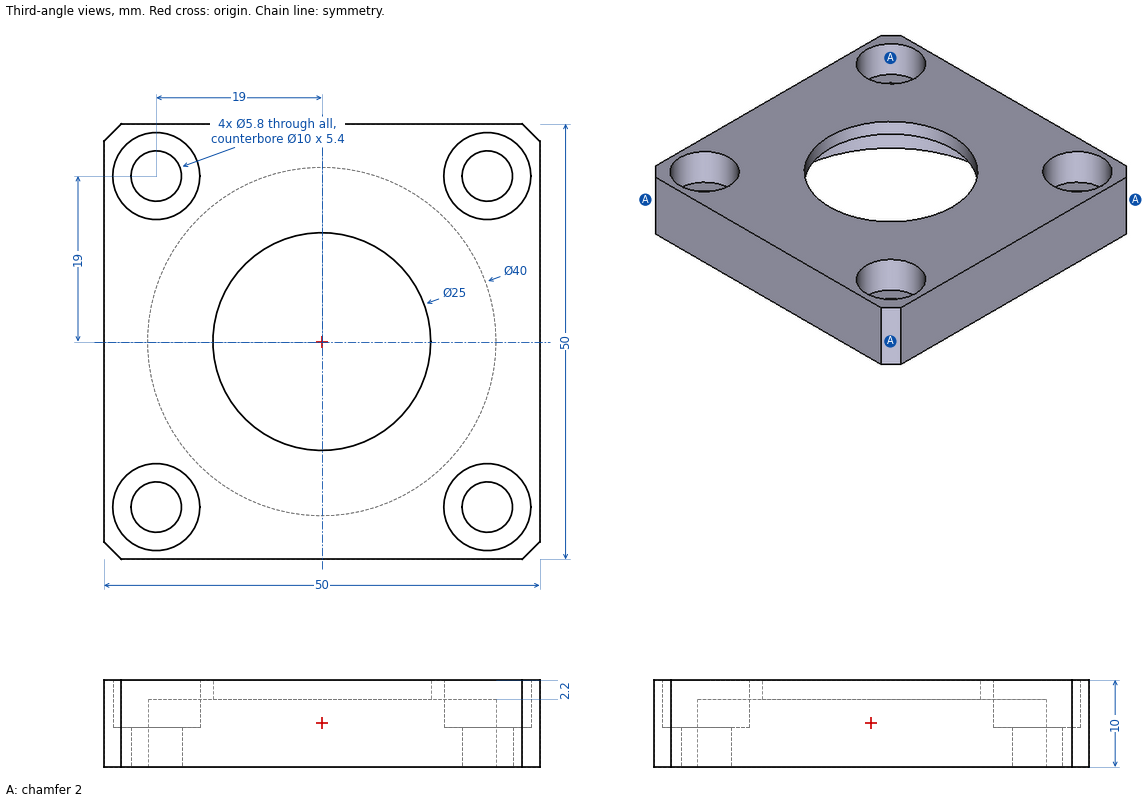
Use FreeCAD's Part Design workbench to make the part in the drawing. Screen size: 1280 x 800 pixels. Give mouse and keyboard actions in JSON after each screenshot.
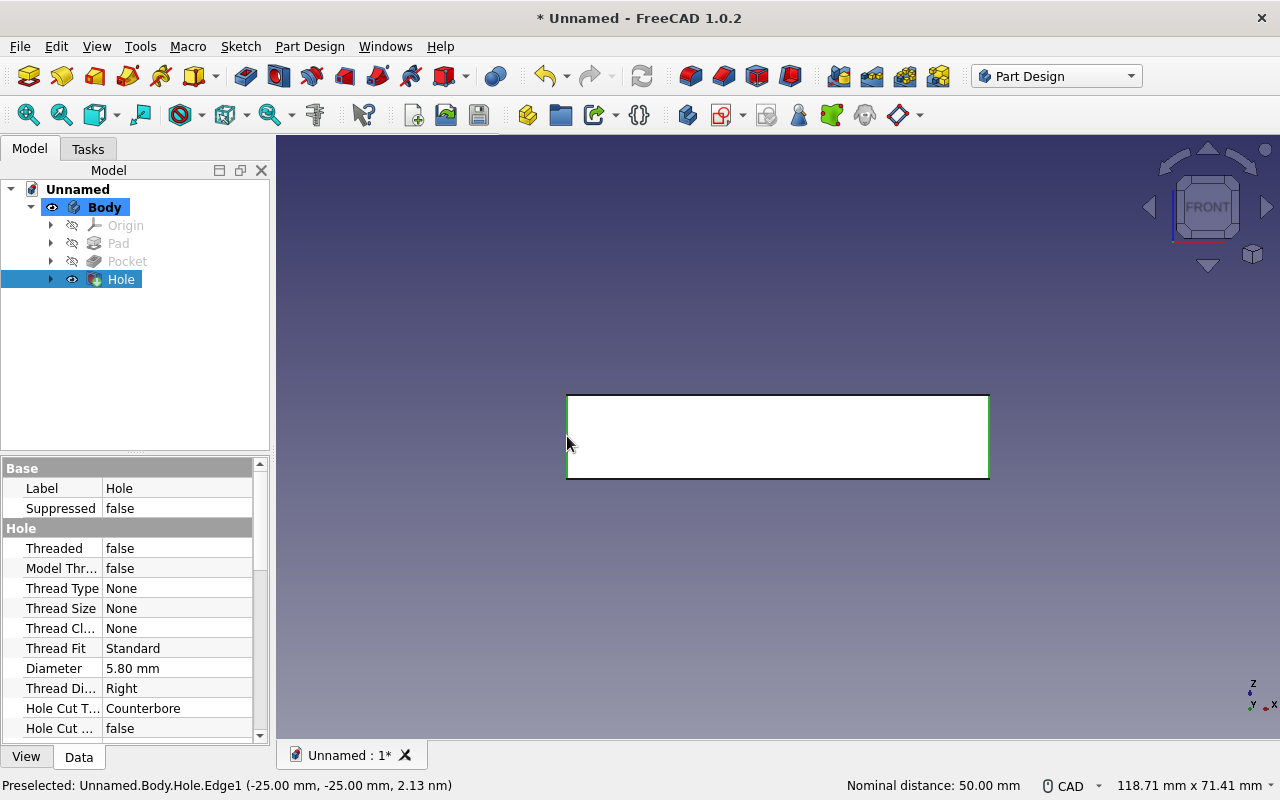
{"action": "key", "text": "3"}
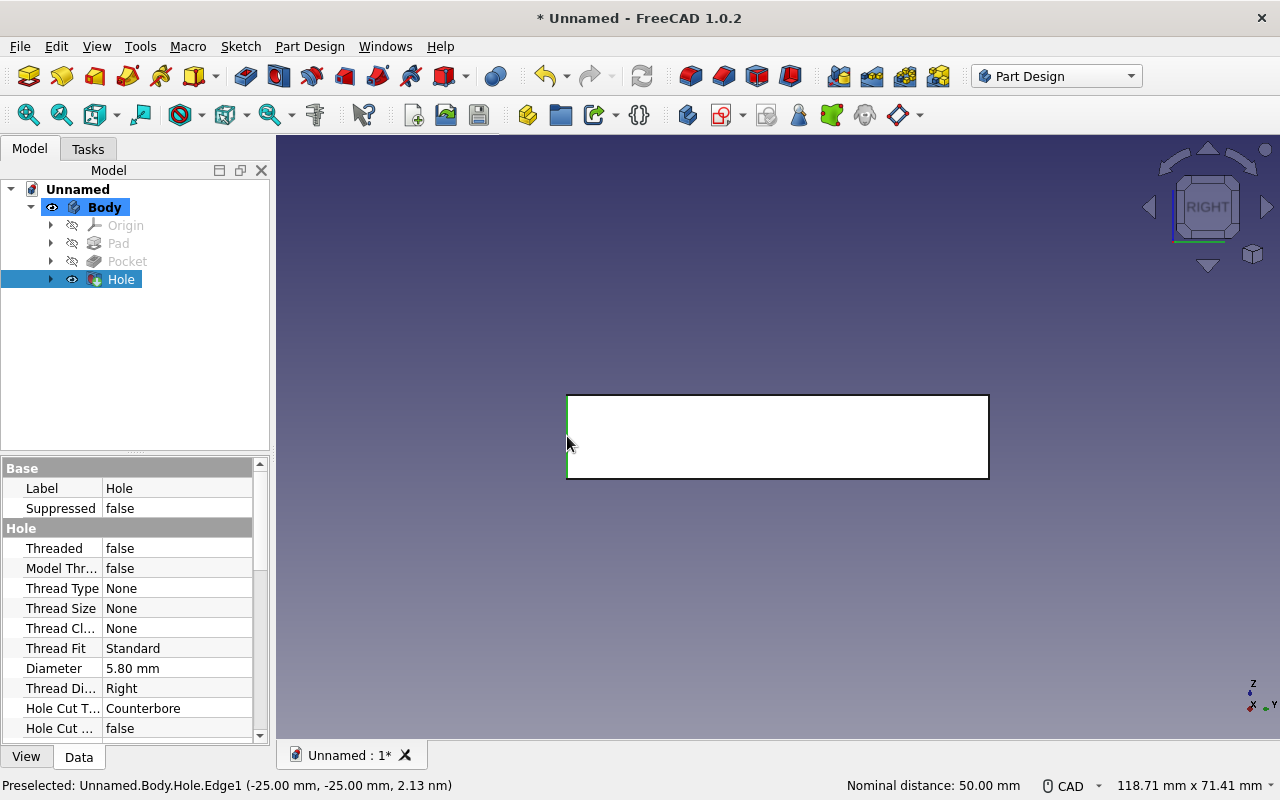
{"action": "left_click", "coordinate": [29, 116]}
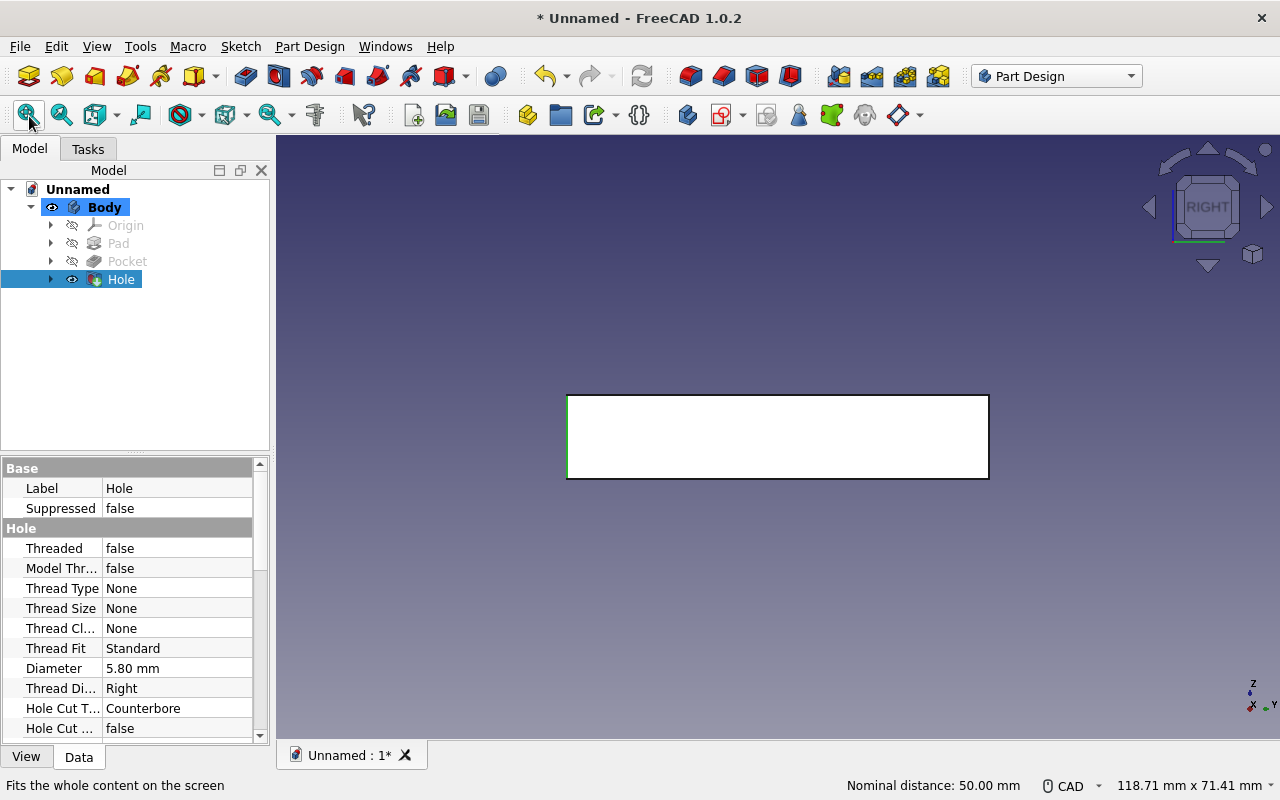
{"action": "left_click", "coordinate": [989, 436], "text": "ctrl"}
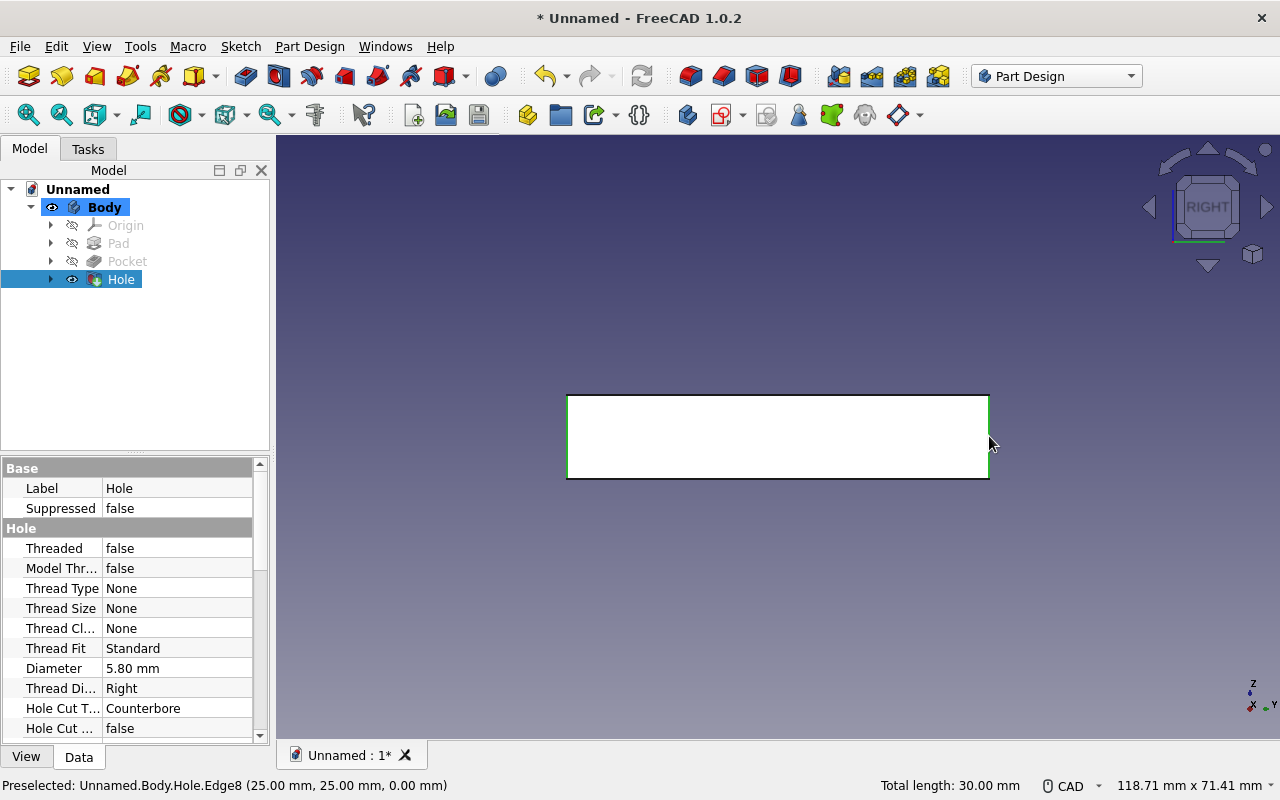
{"action": "key", "text": "5"}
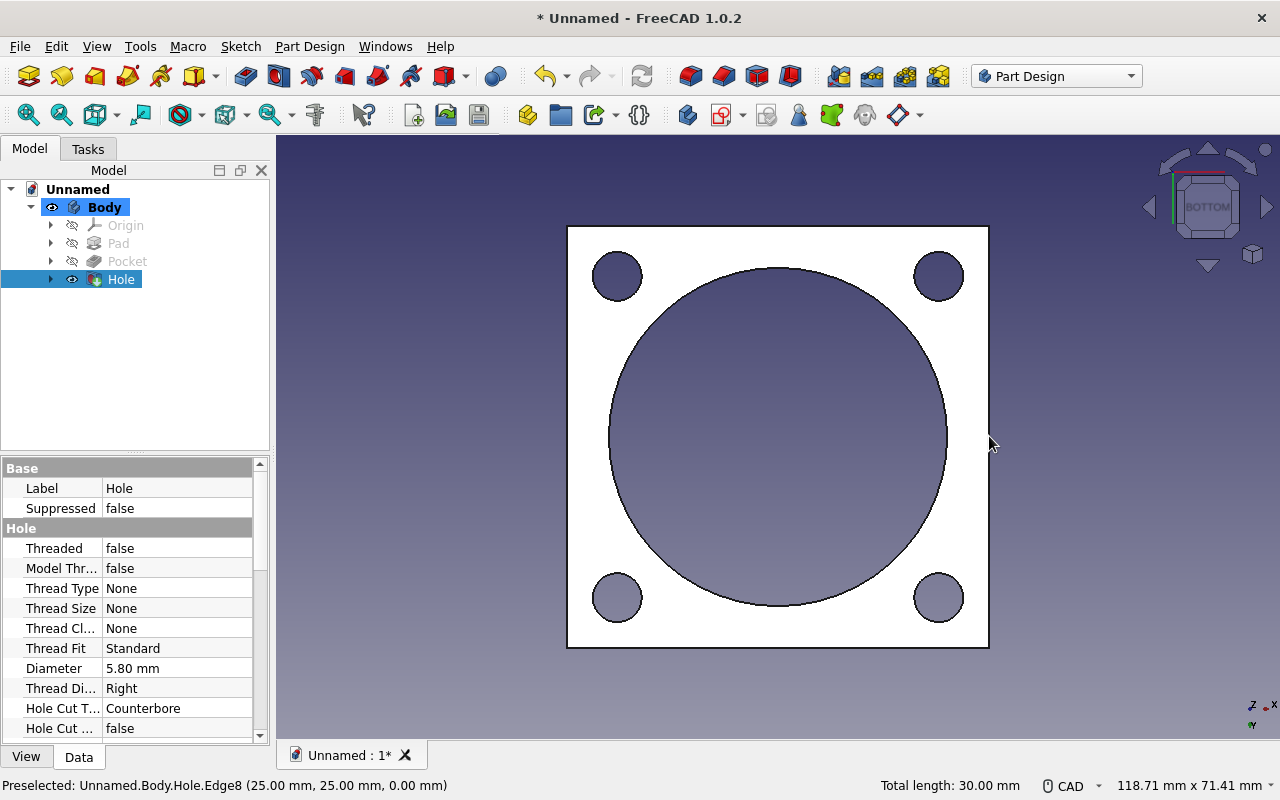
{"action": "key", "text": "4"}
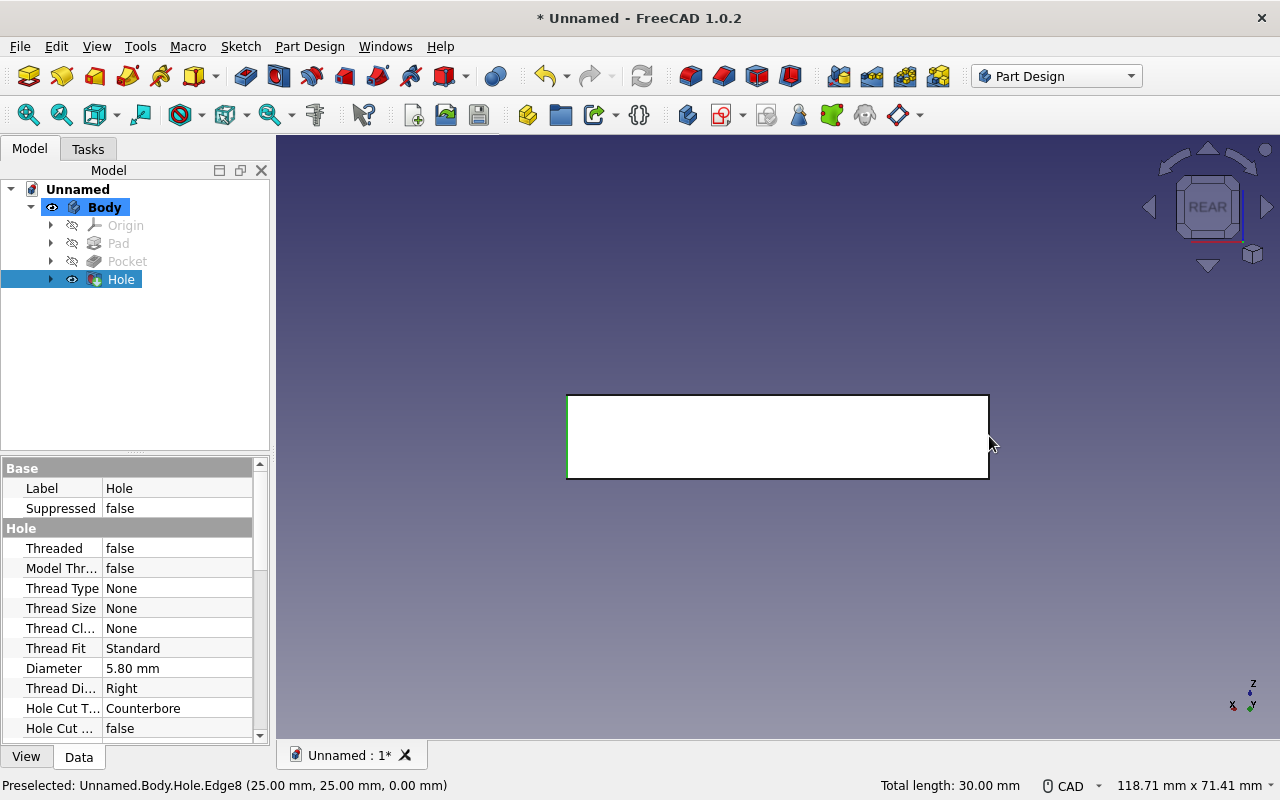
{"action": "left_click", "coordinate": [29, 116]}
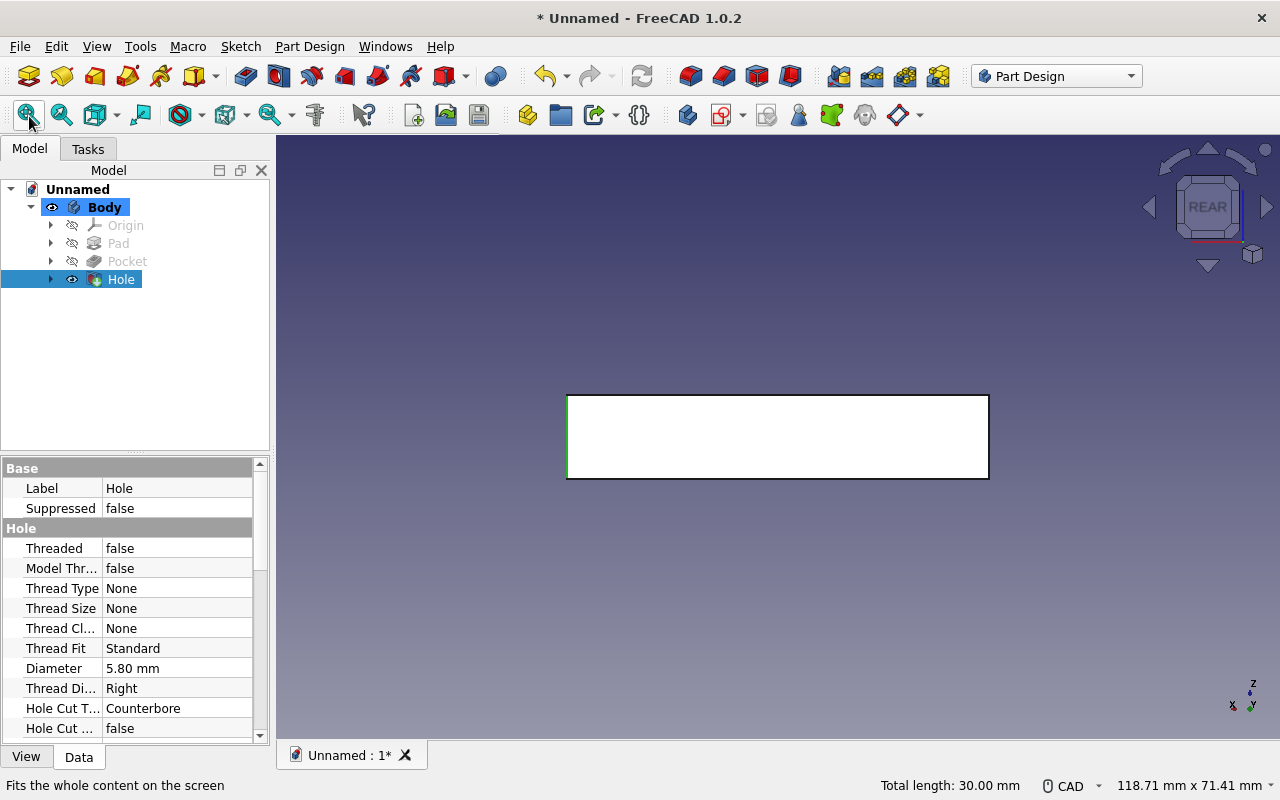
{"action": "left_click", "coordinate": [989, 436], "text": "ctrl"}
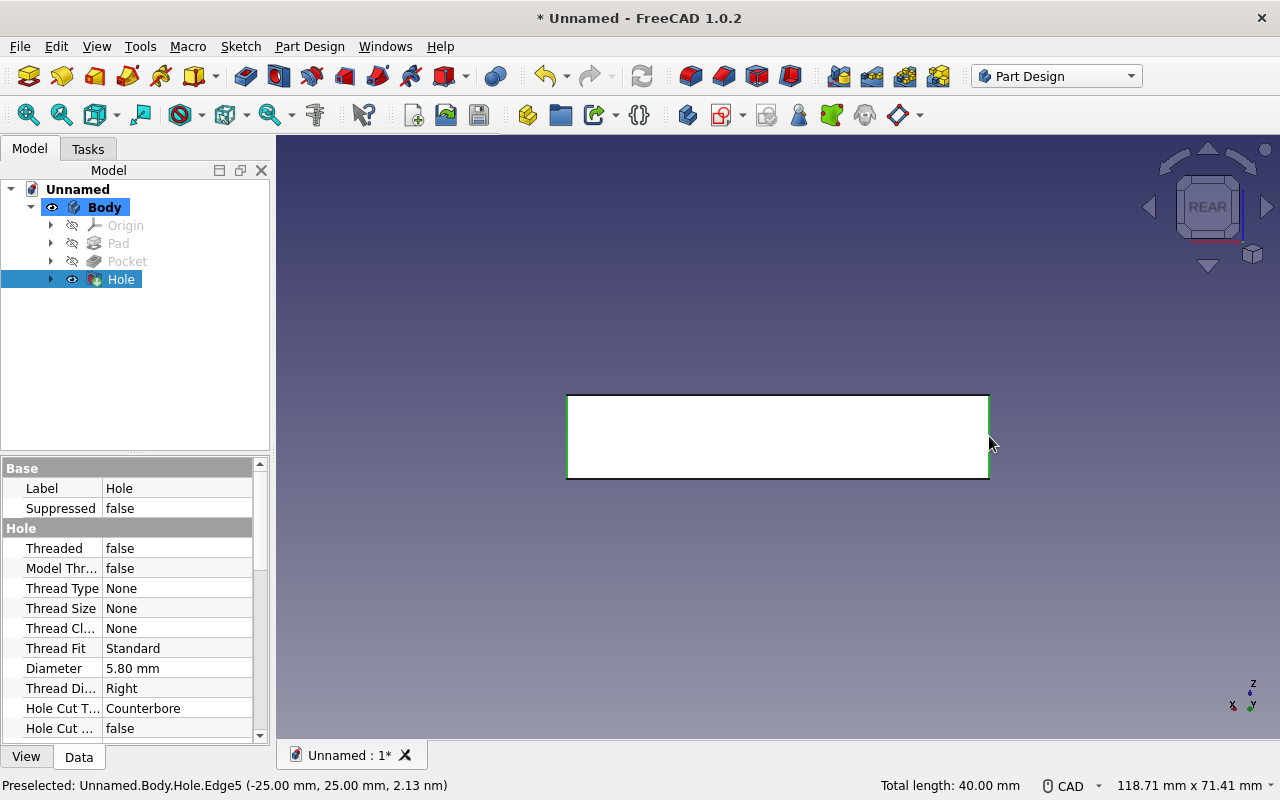
{"action": "left_click", "coordinate": [724, 76]}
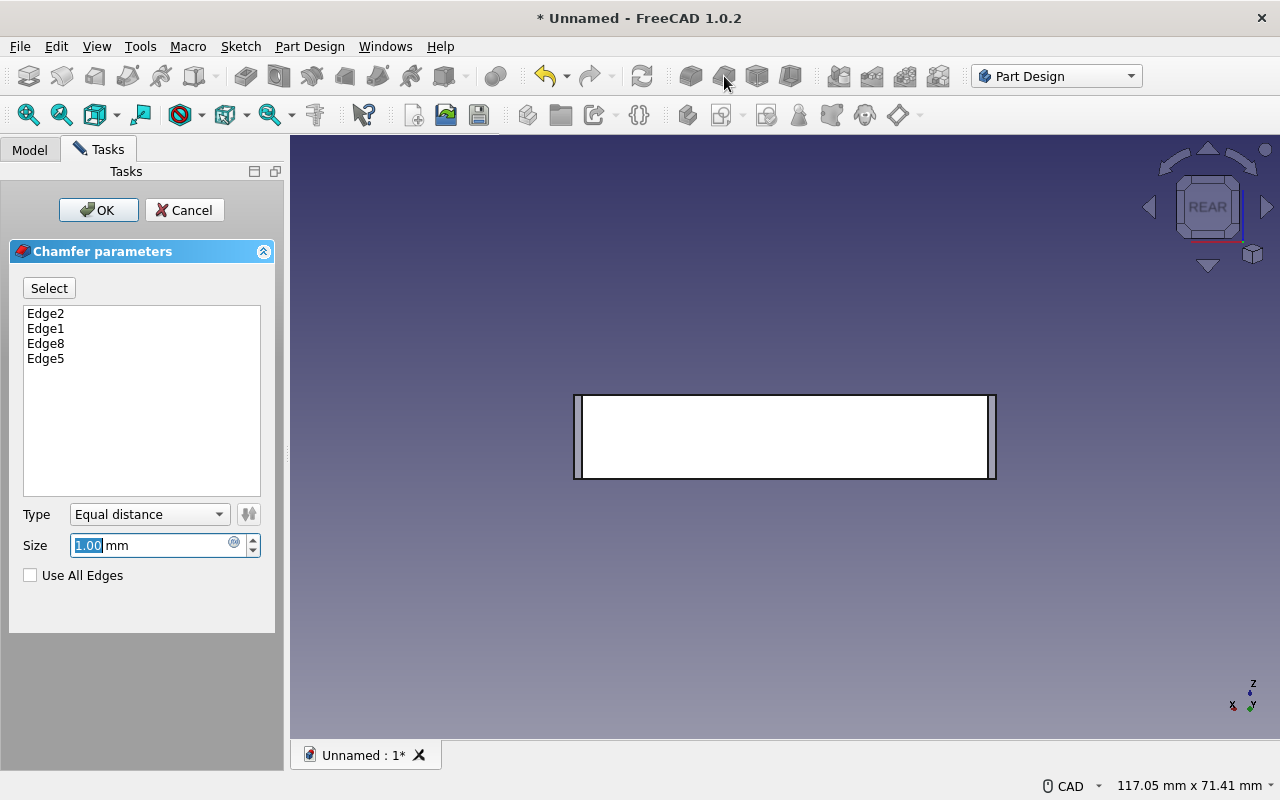
{"action": "type", "text": "2"}
{"action": "key", "text": "Tab"}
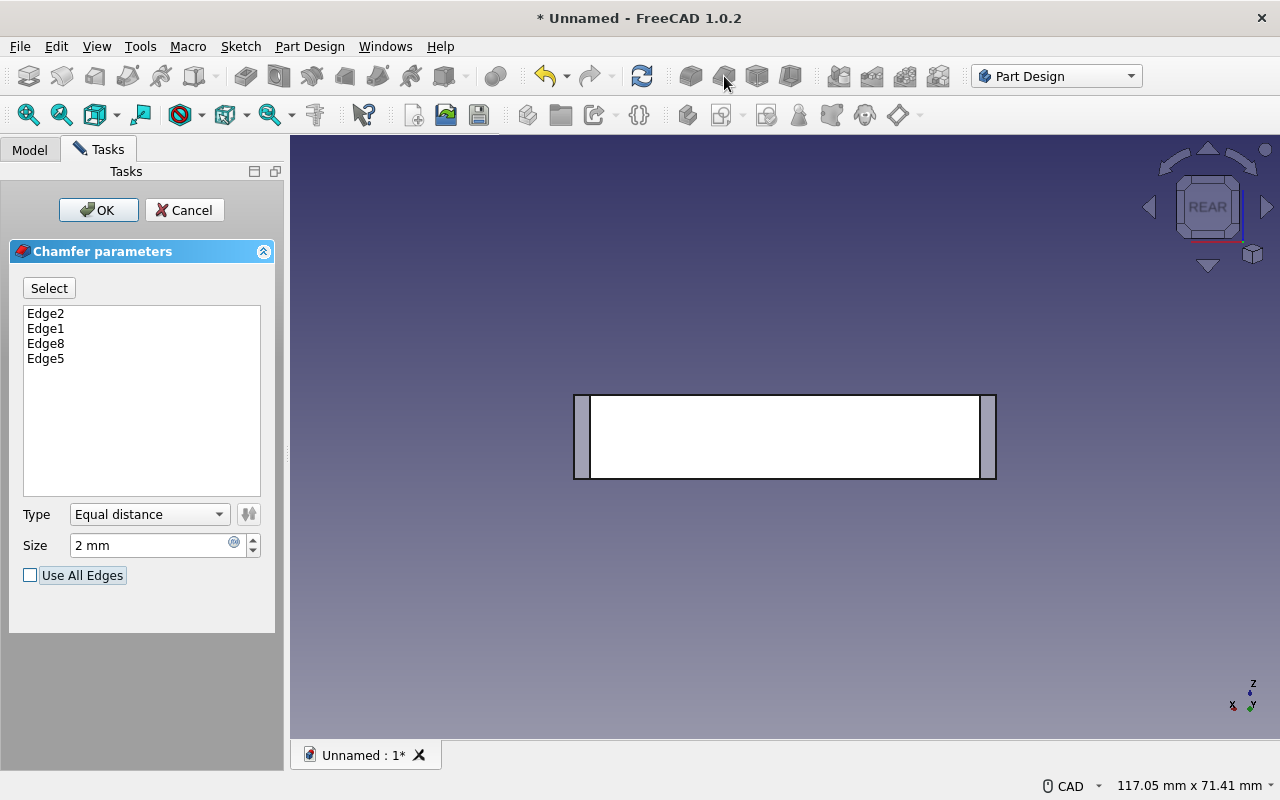
{"action": "left_click", "coordinate": [99, 210]}